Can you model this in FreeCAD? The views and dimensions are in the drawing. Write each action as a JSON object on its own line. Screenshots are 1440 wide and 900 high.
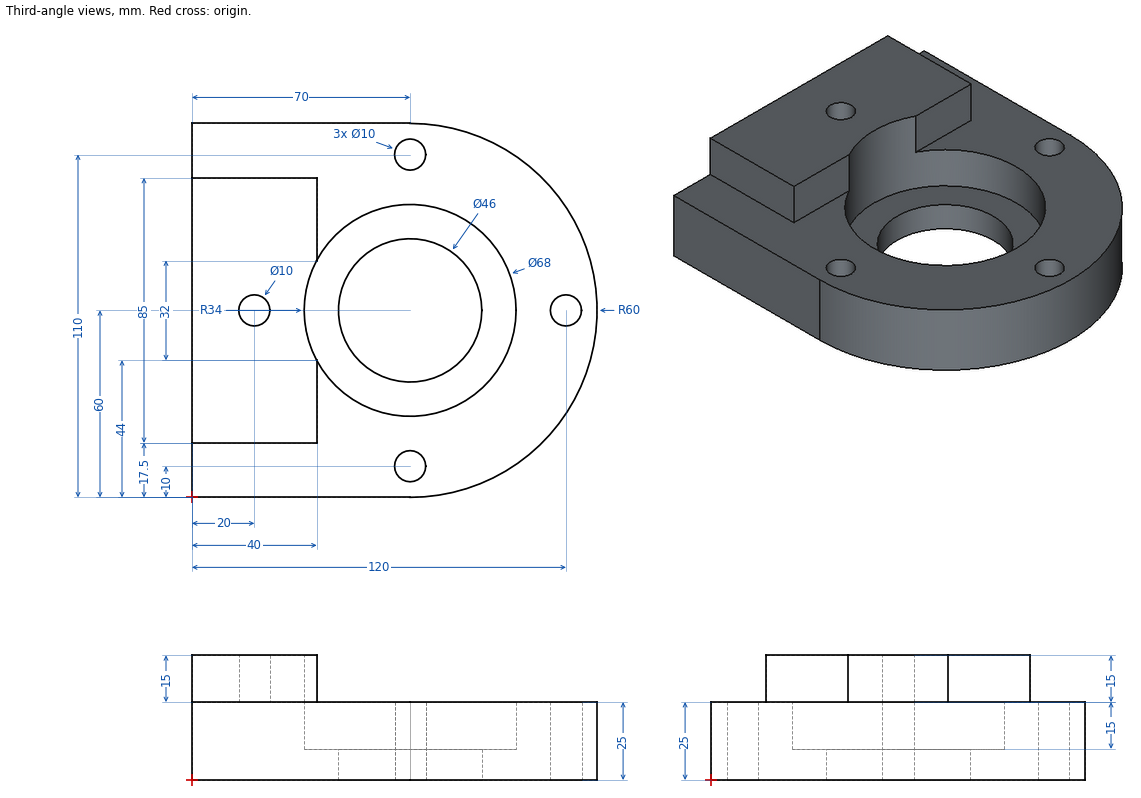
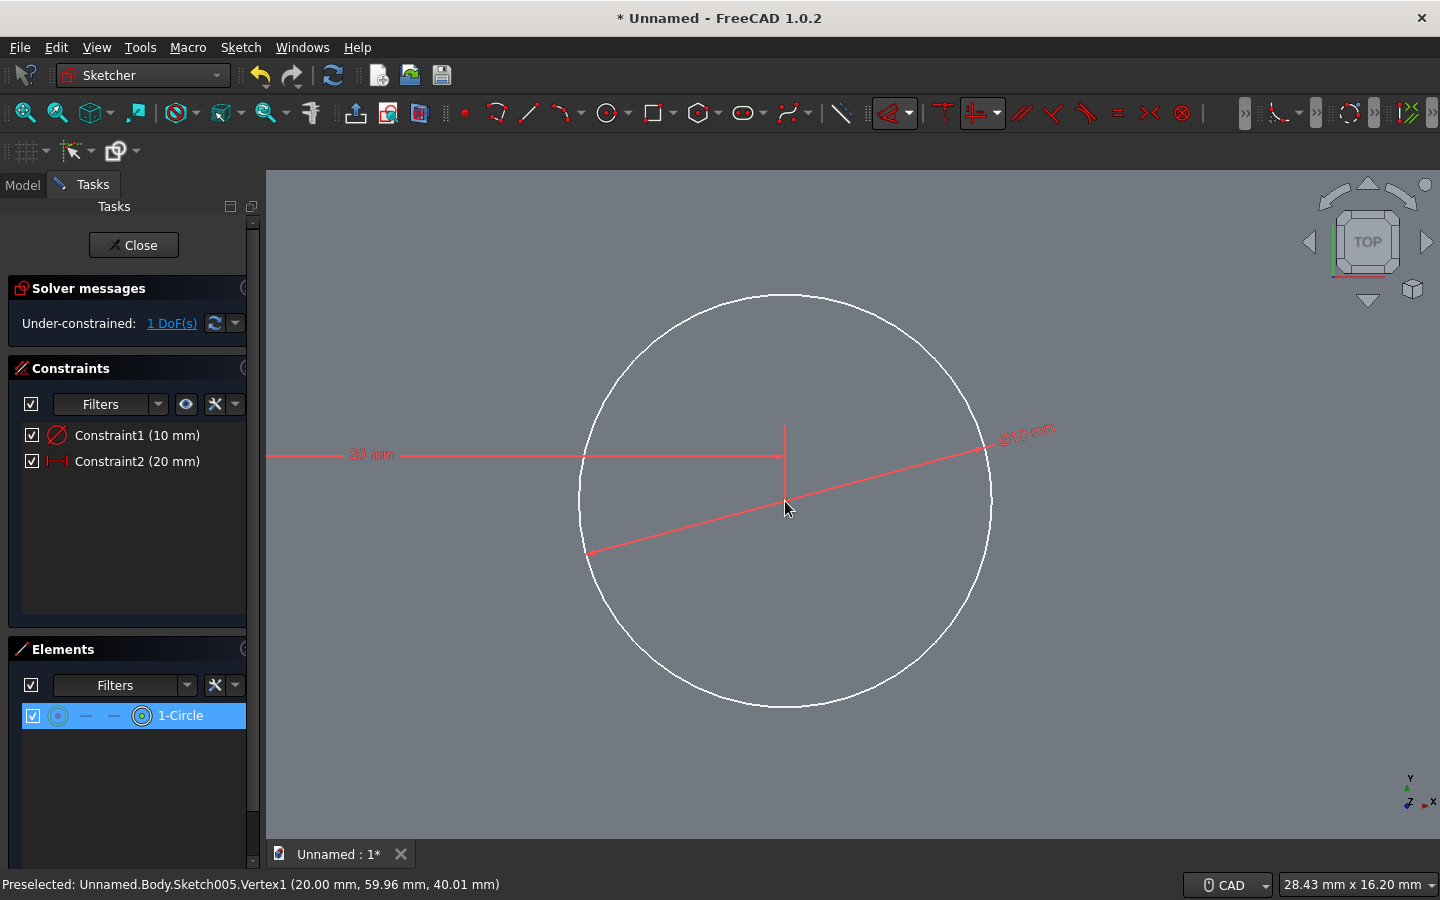
{"action": "key", "text": "i"}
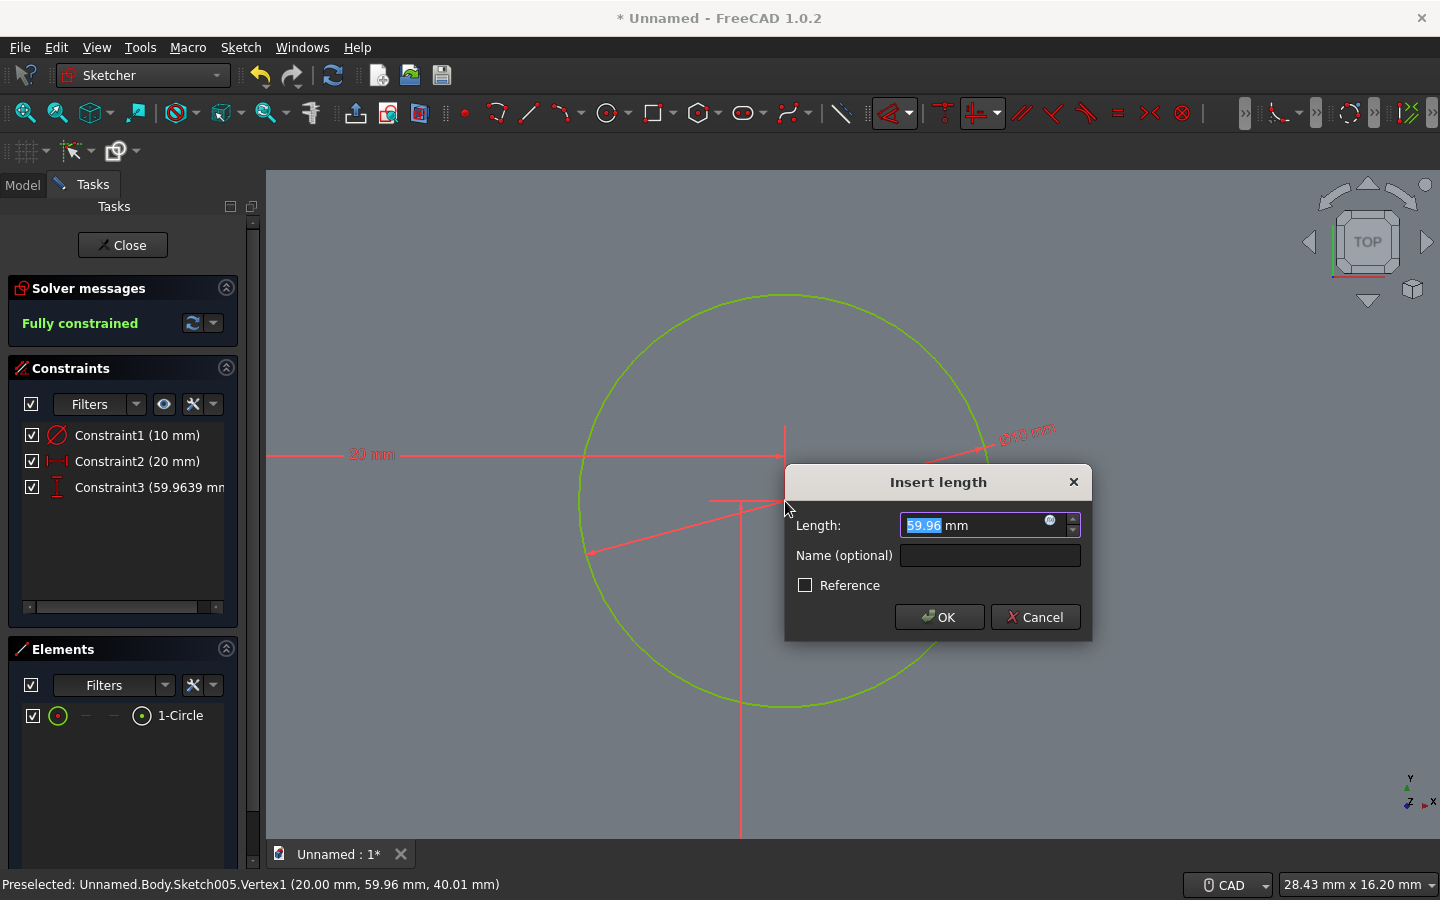
{"action": "type", "text": "60"}
{"action": "key", "text": "Return"}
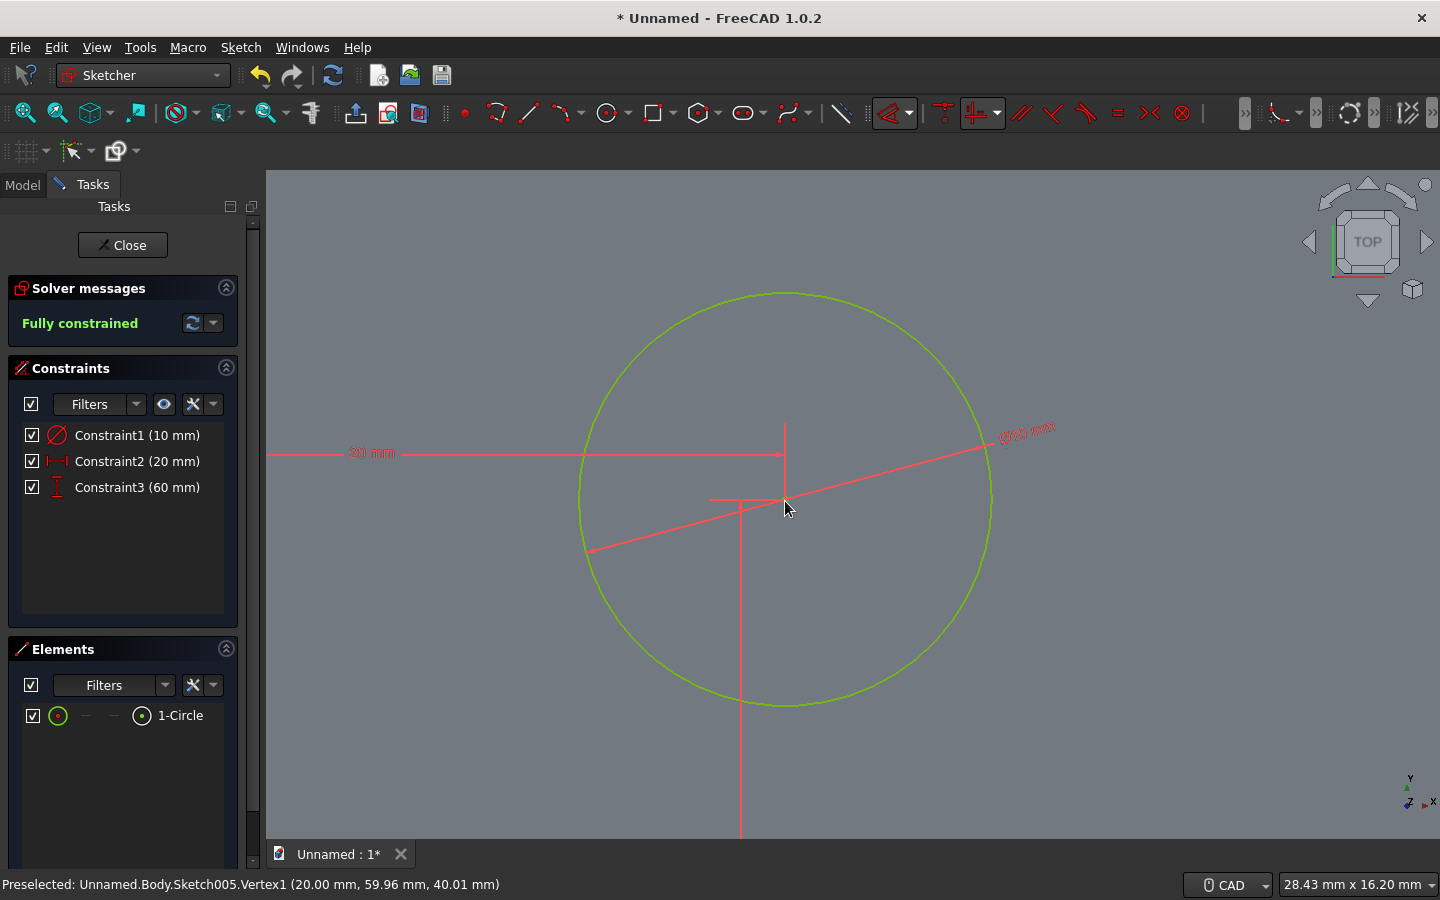
{"action": "left_click", "coordinate": [123, 245]}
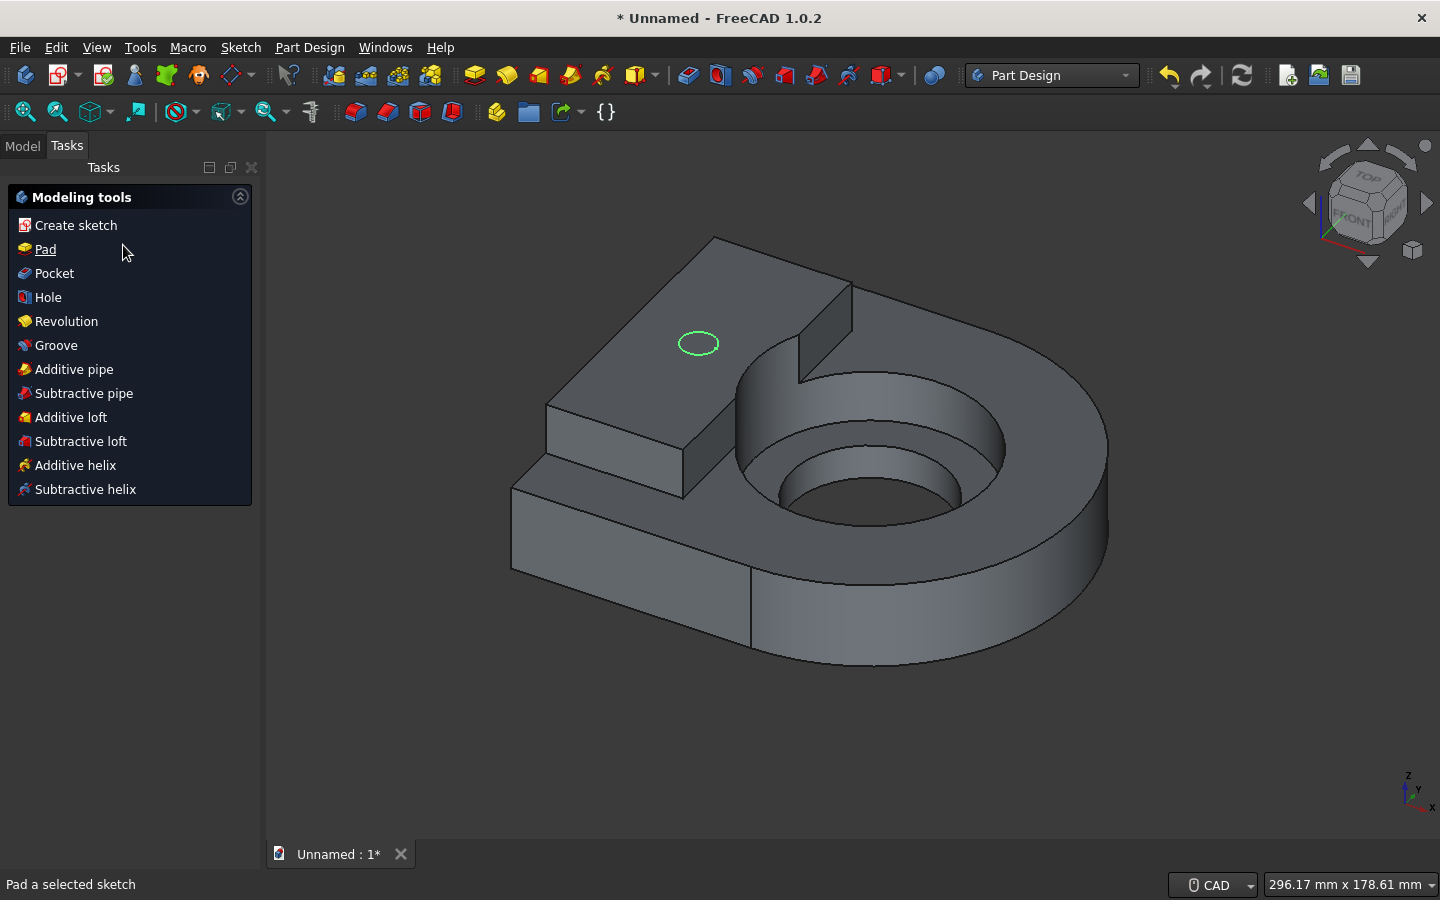
{"action": "left_click", "coordinate": [690, 76]}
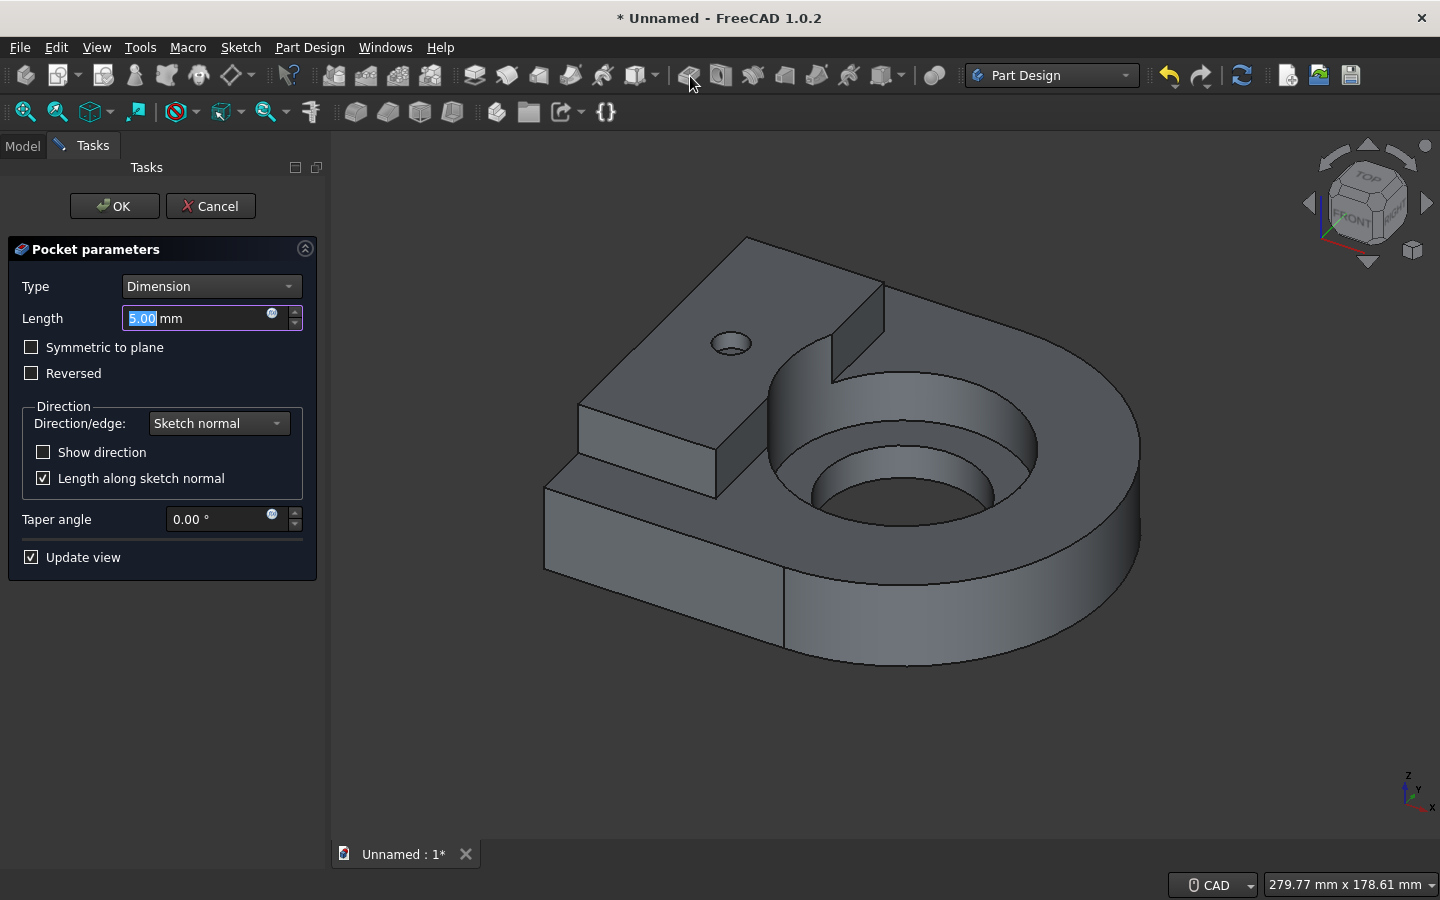
{"action": "type", "text": "15"}
{"action": "key", "text": "Tab"}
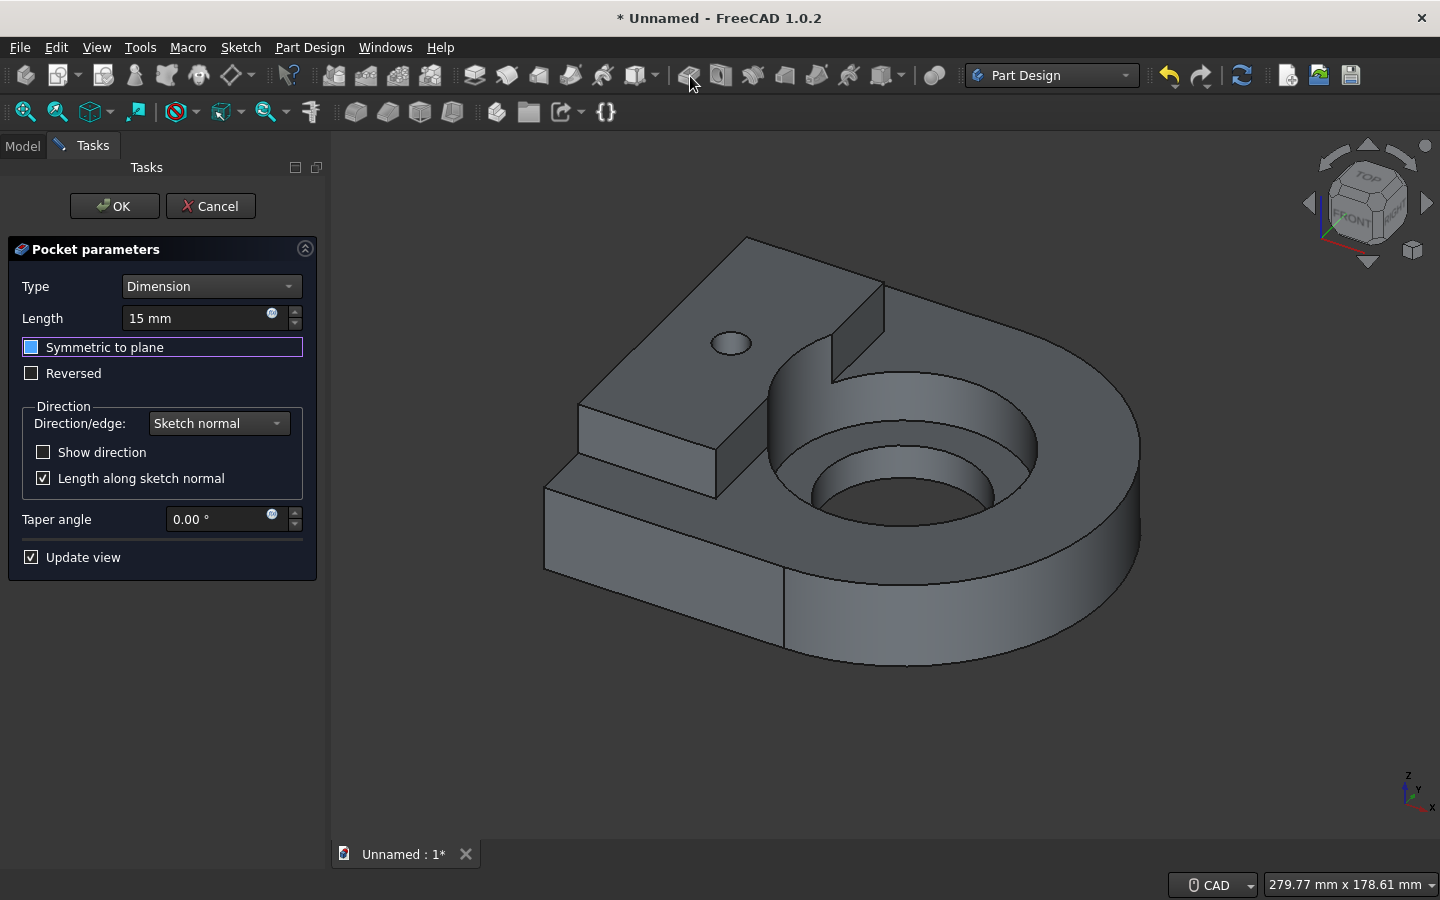
{"action": "left_click", "coordinate": [115, 206]}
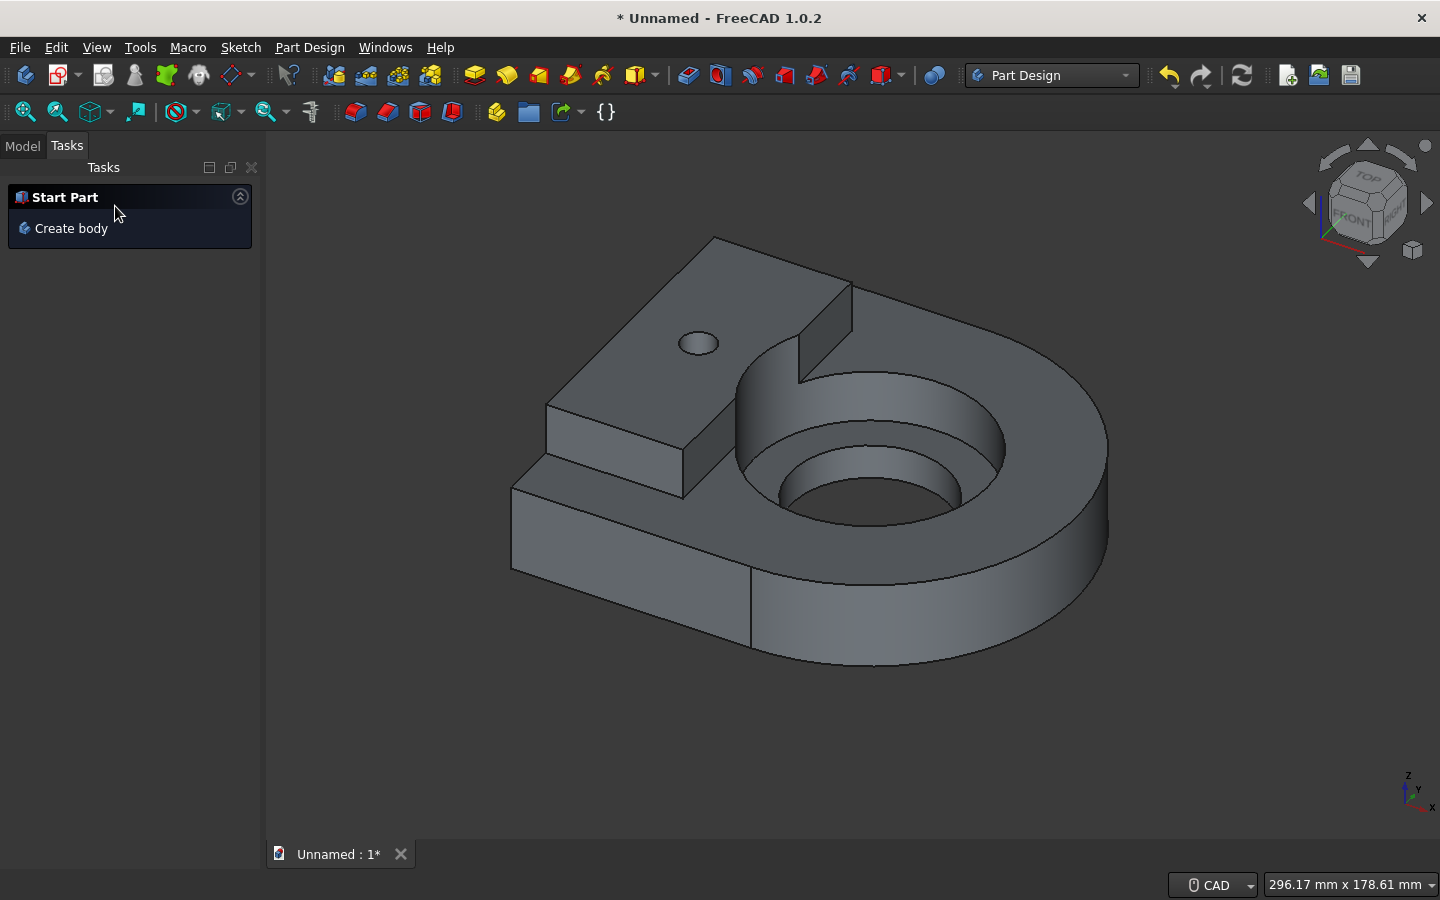
{"action": "left_click", "coordinate": [1049, 417]}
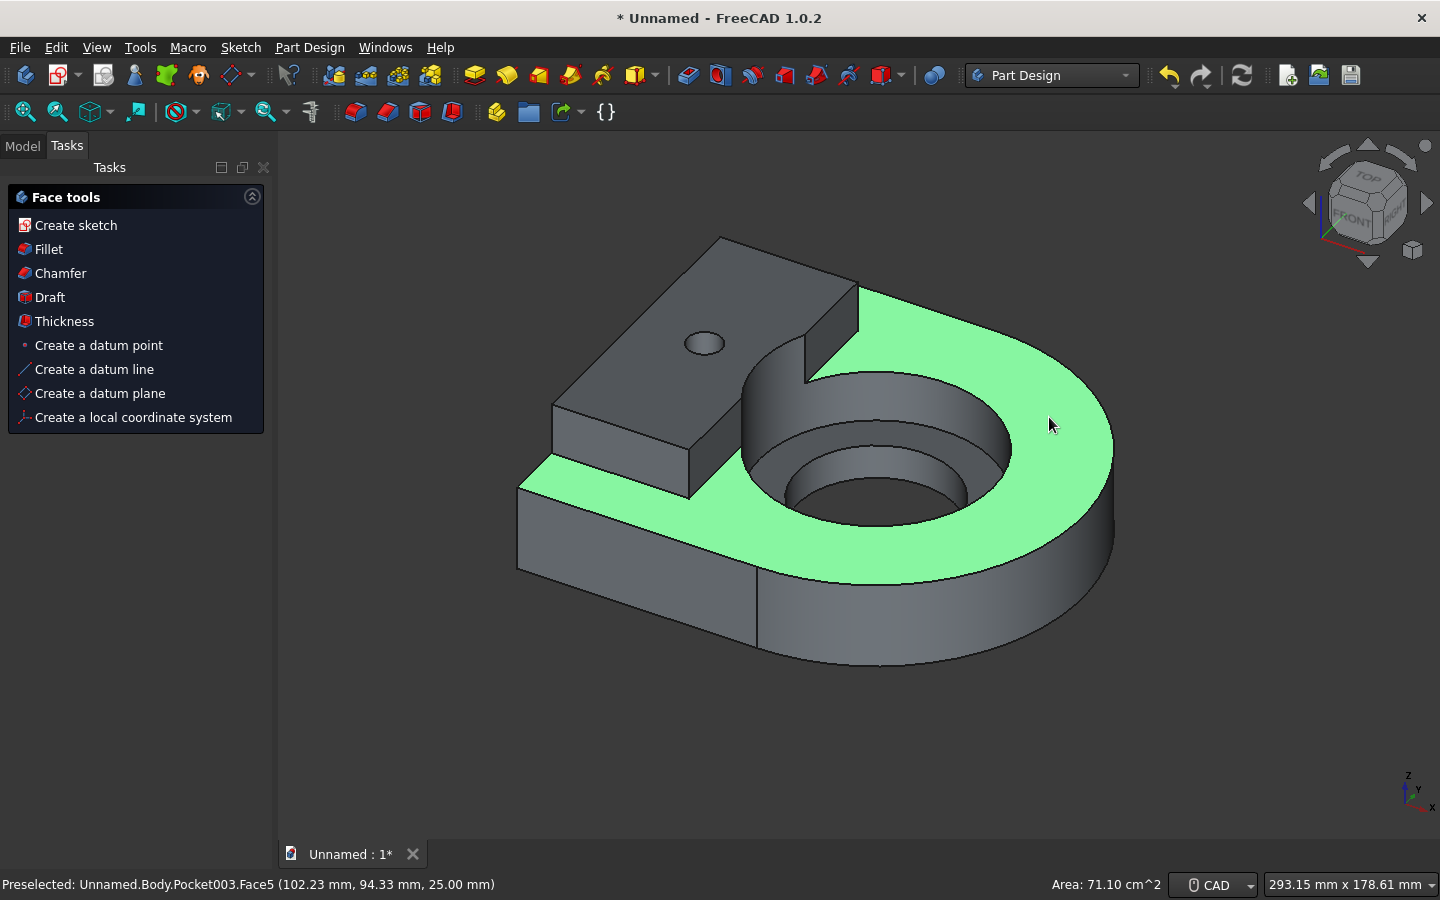
{"action": "left_click", "coordinate": [58, 76]}